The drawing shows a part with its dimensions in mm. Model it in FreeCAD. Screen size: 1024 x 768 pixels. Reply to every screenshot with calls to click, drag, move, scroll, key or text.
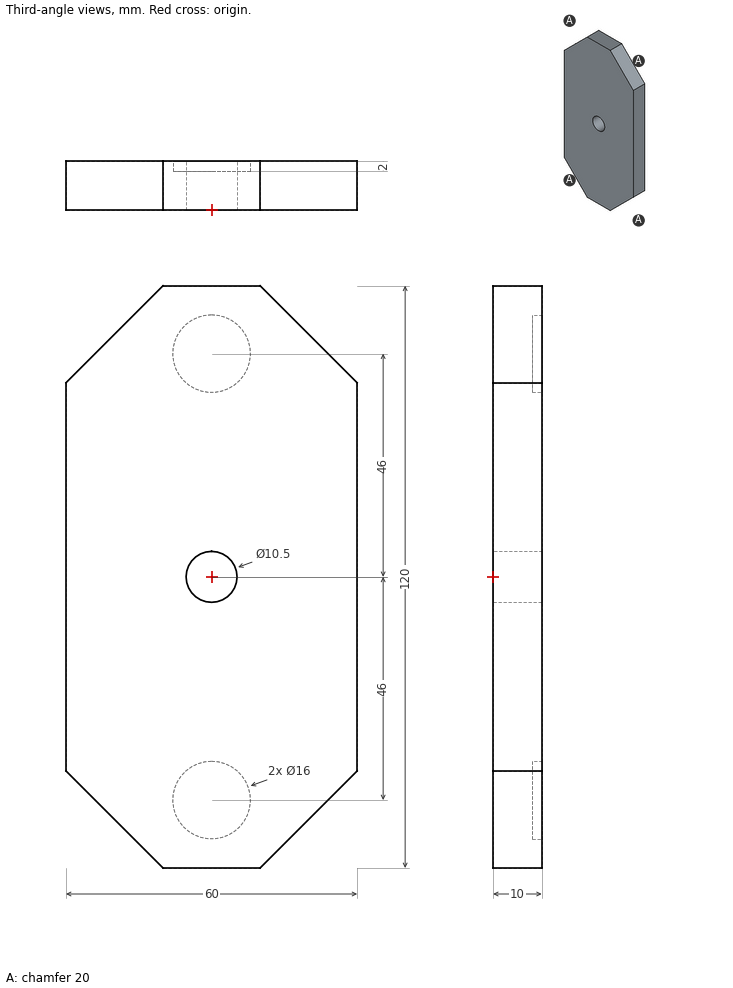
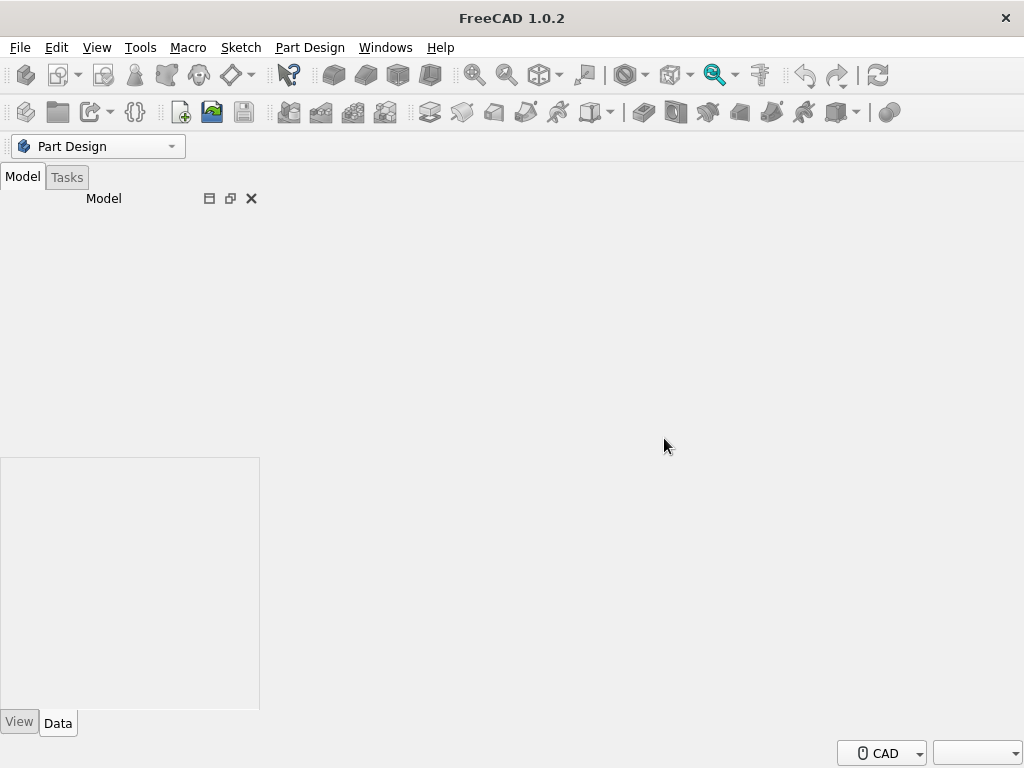
click(180, 112)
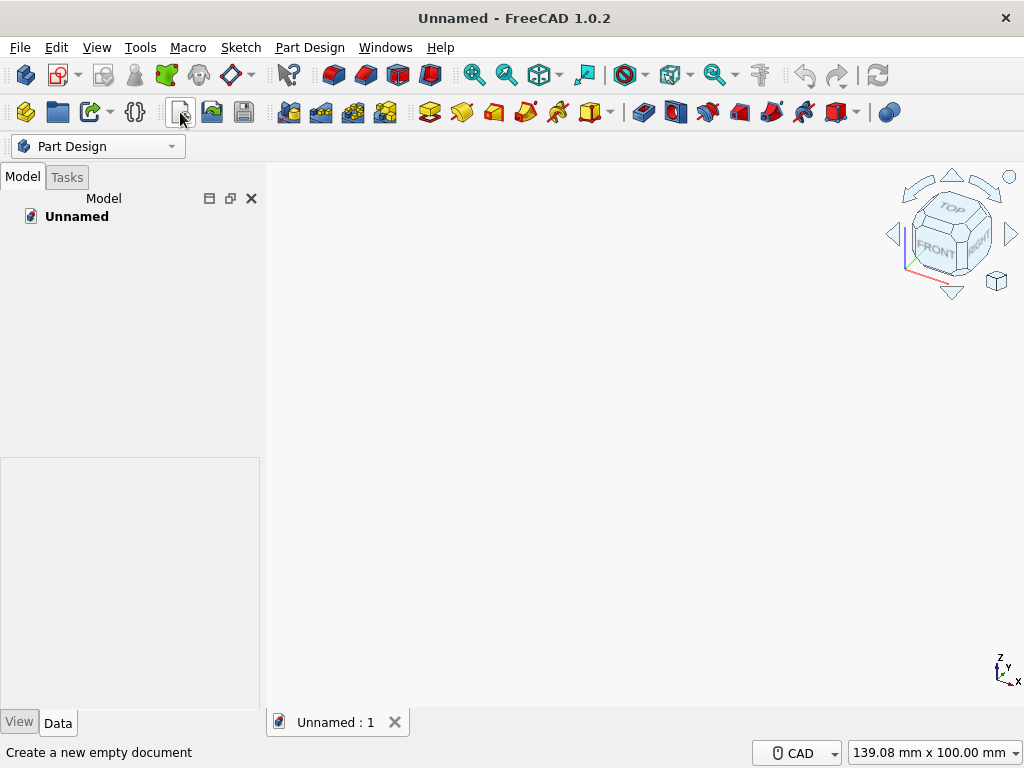
click(58, 76)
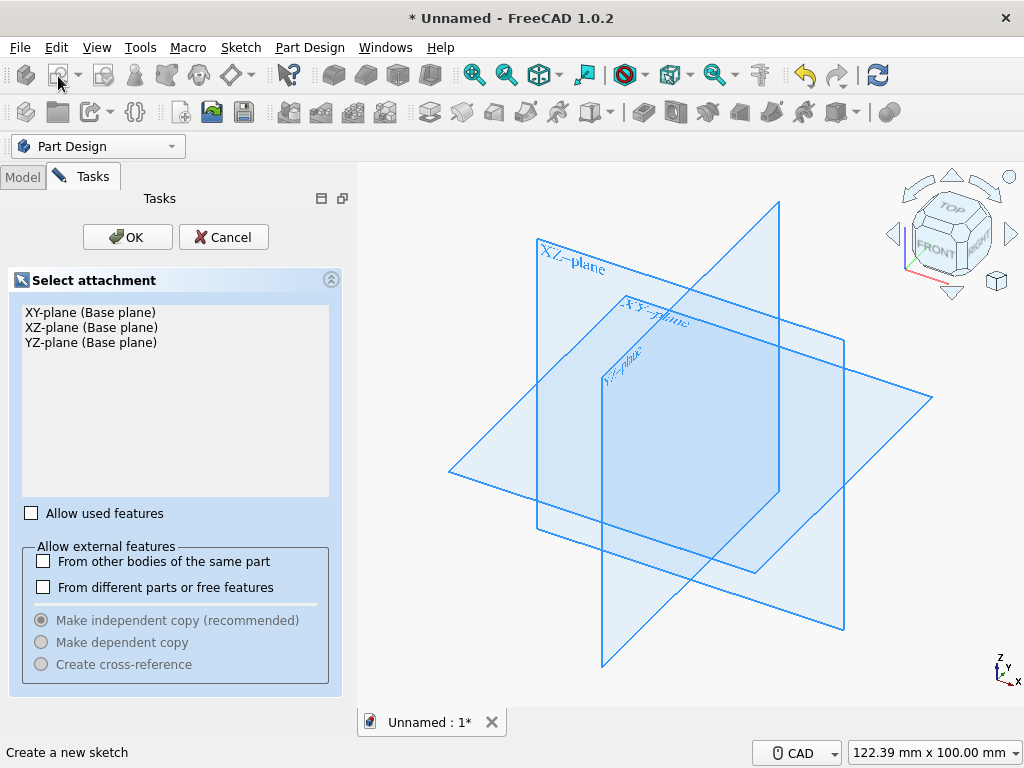
click(82, 328)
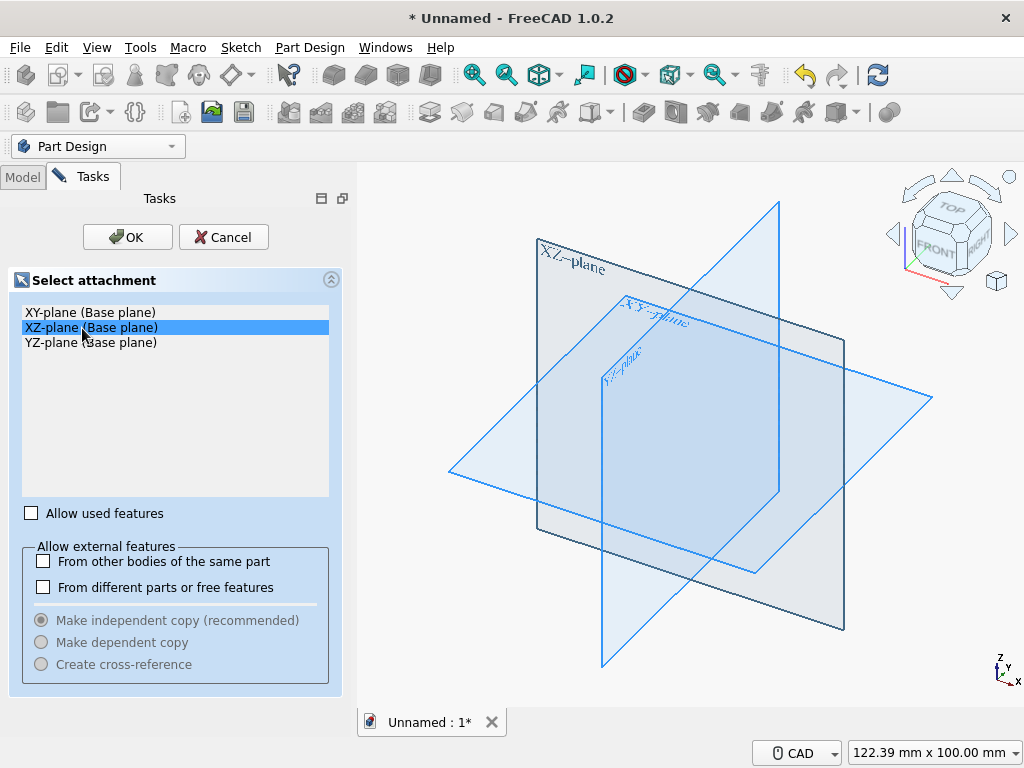
click(128, 237)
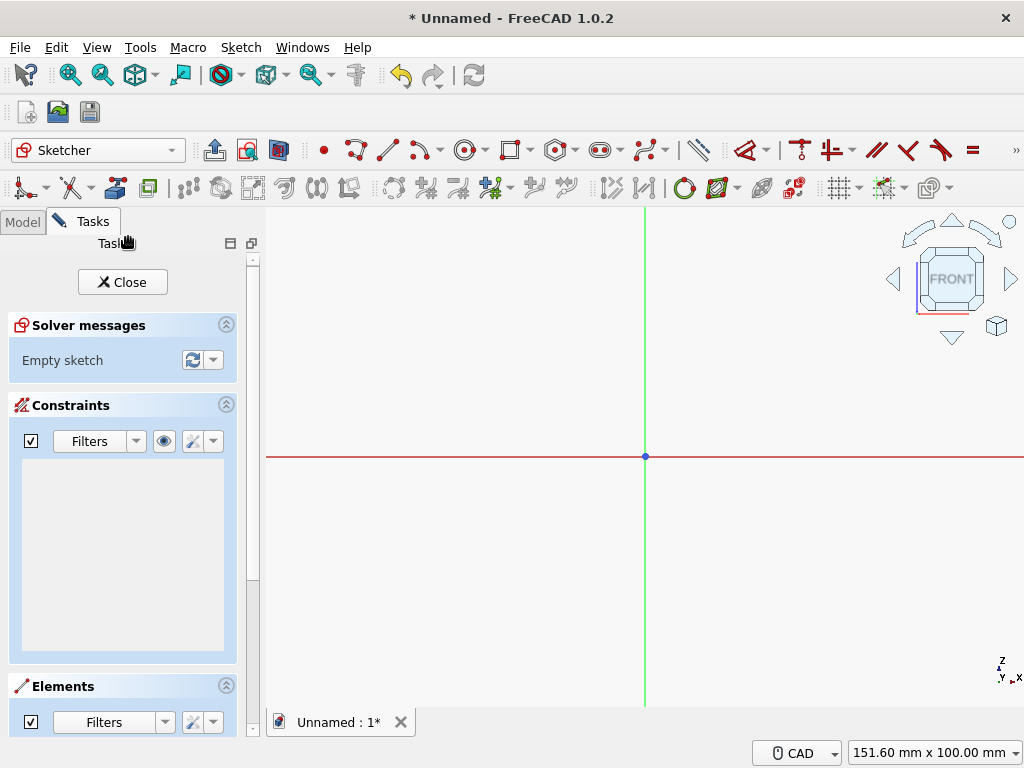
scroll(493, 457, down, 3)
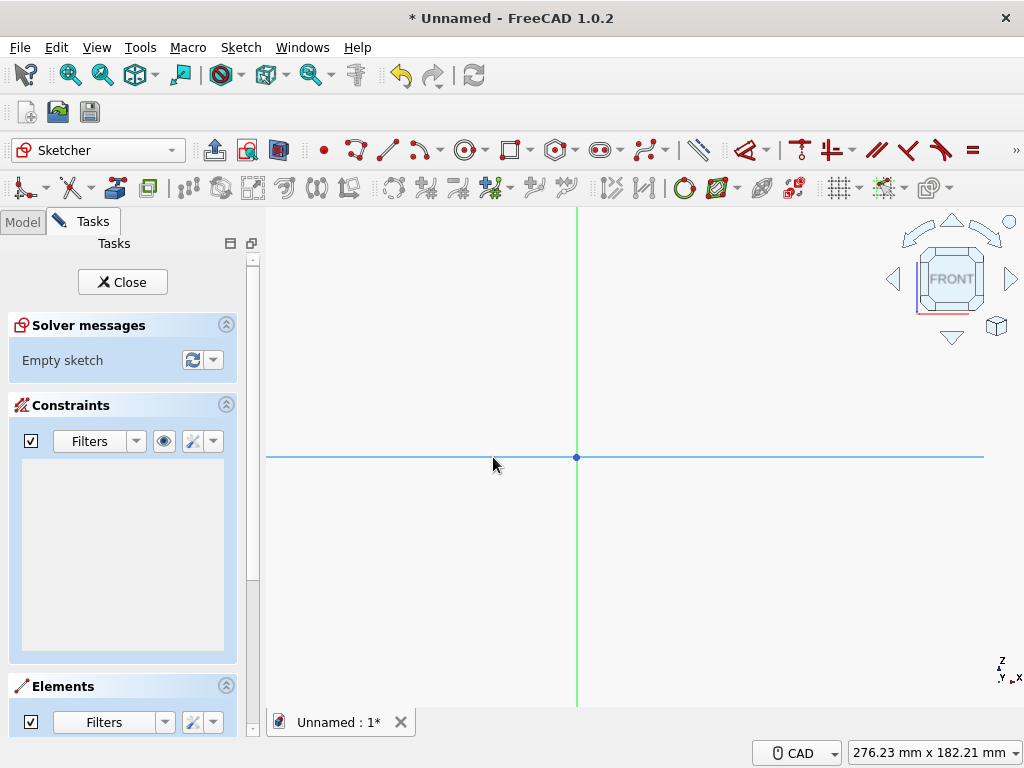
click(532, 150)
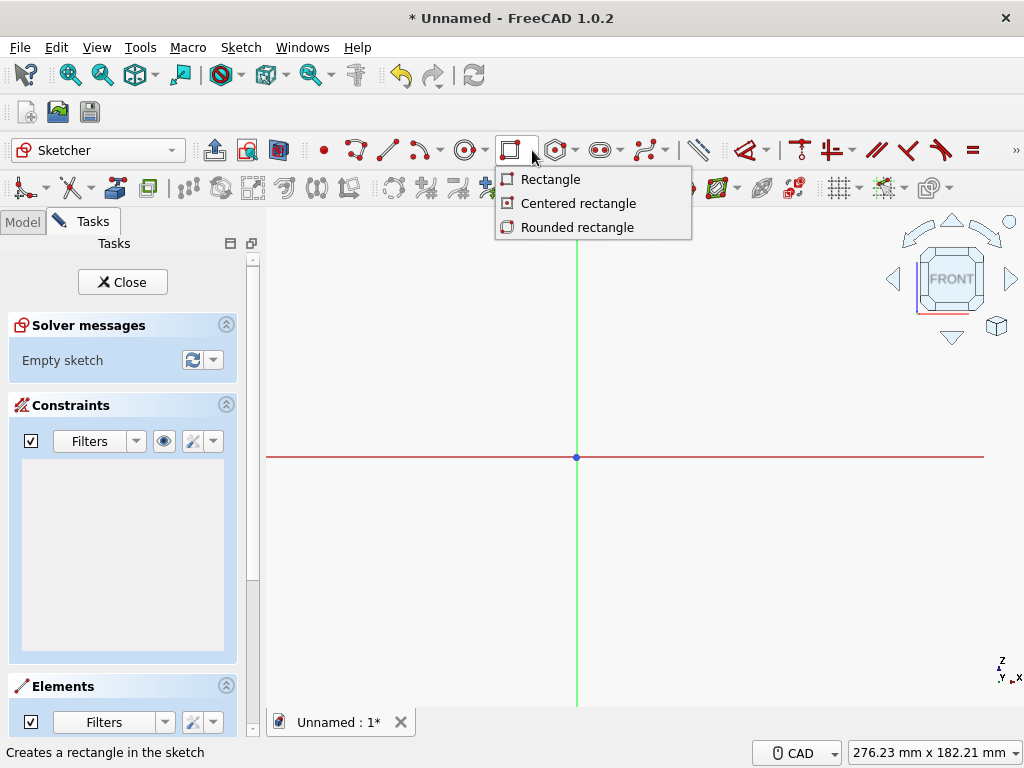
click(594, 203)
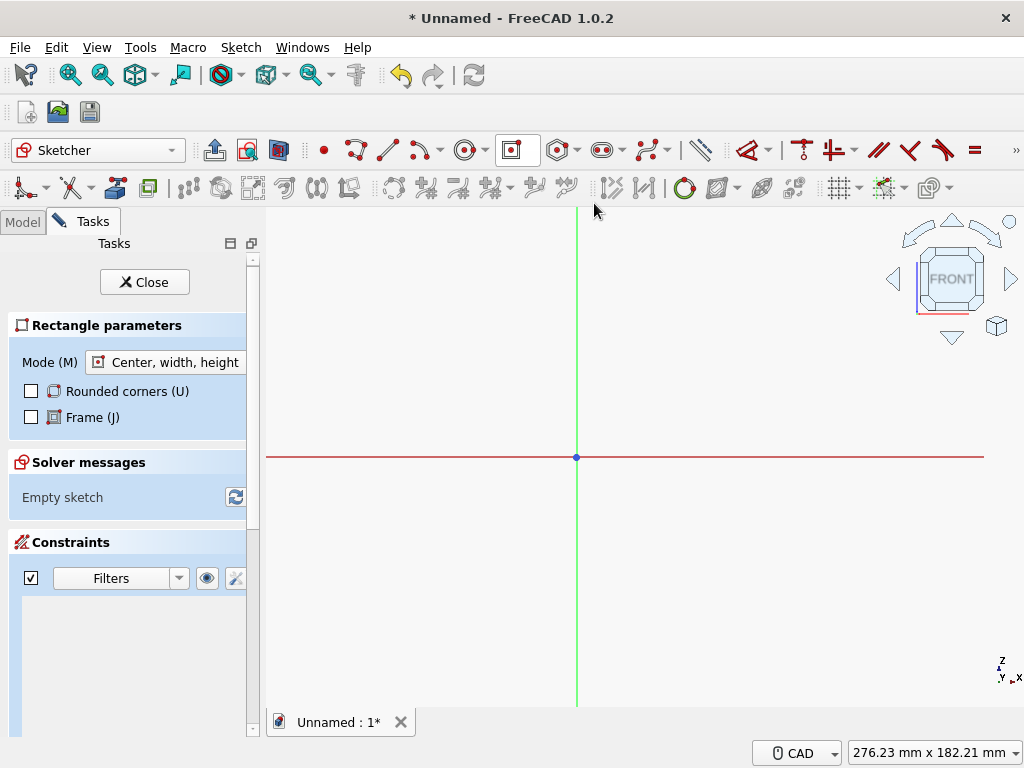
click(577, 457)
click(659, 293)
key(Escape)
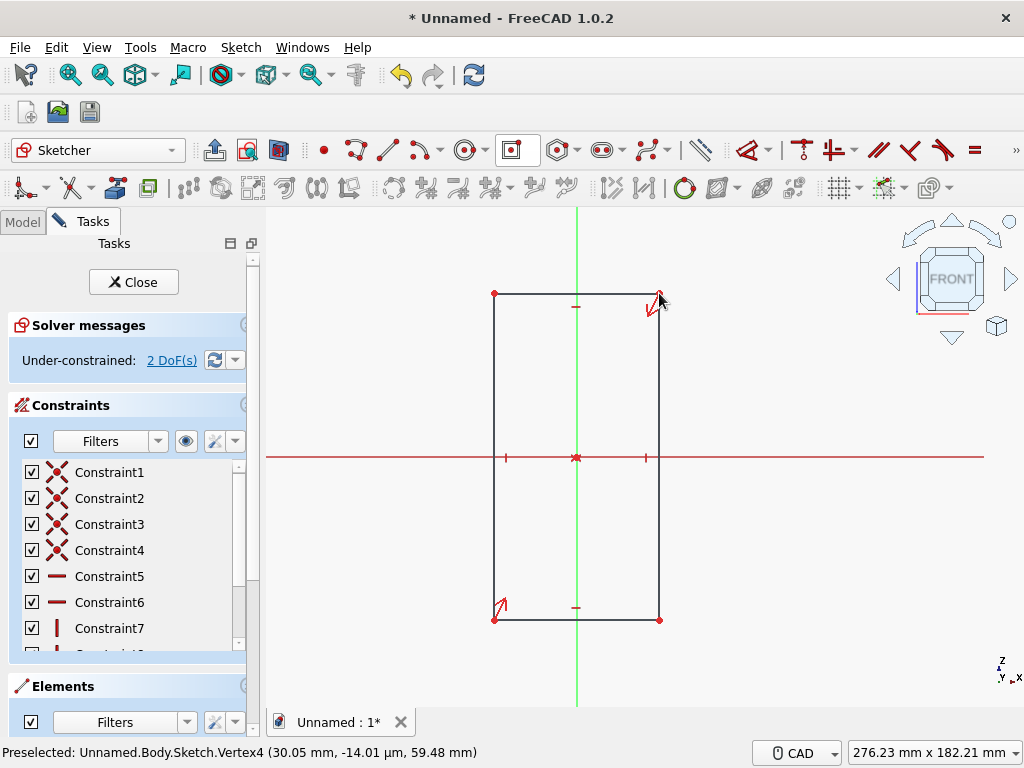
click(748, 150)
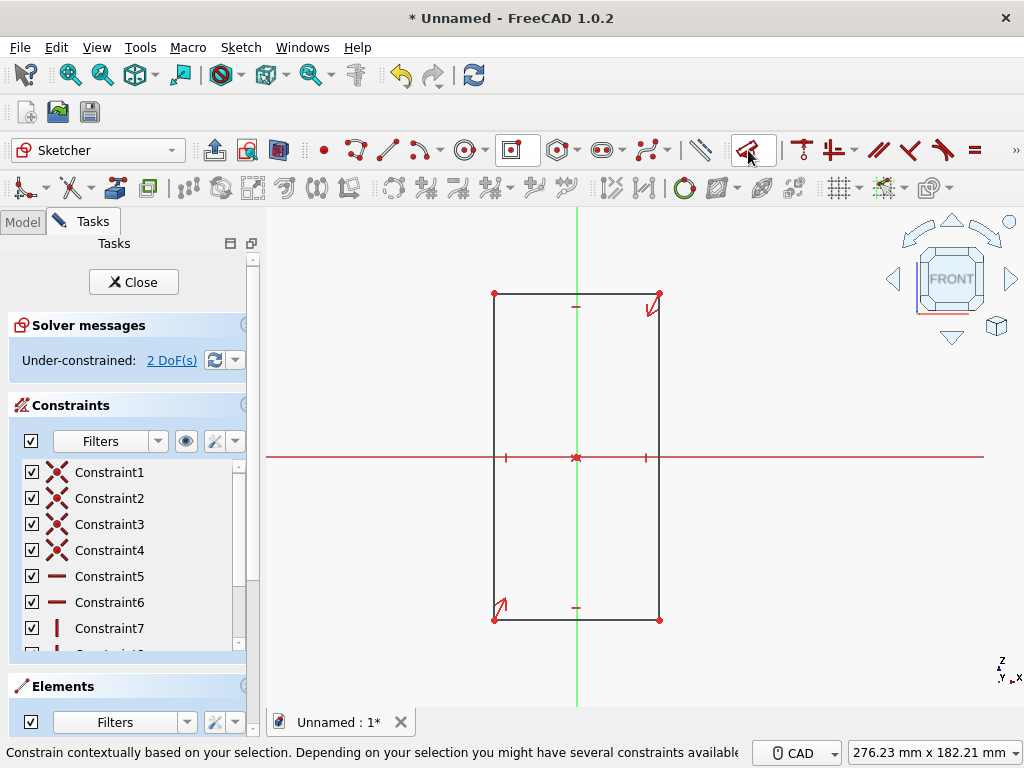
click(544, 620)
click(539, 654)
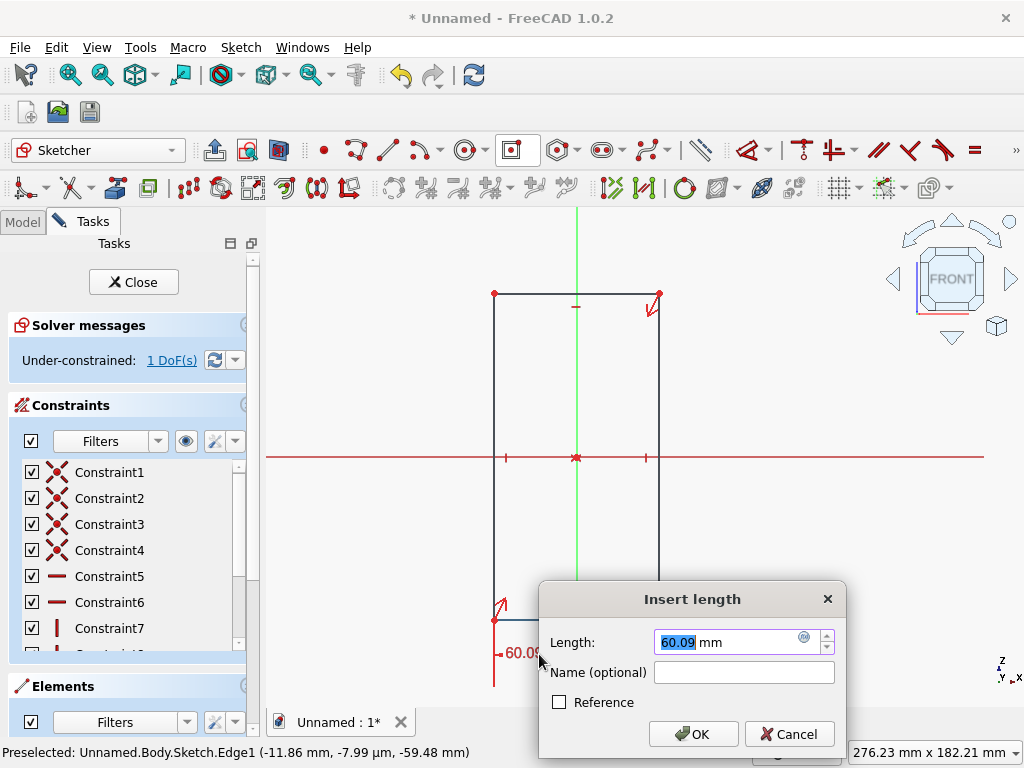
text(60)
key(Return)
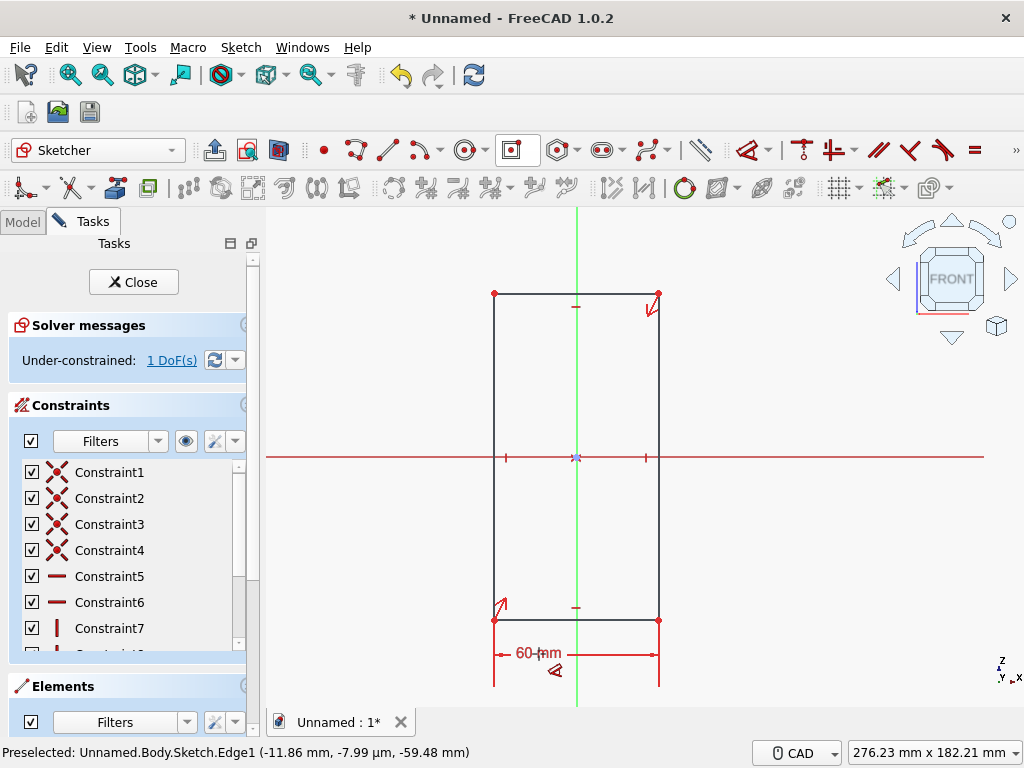
click(659, 523)
click(693, 382)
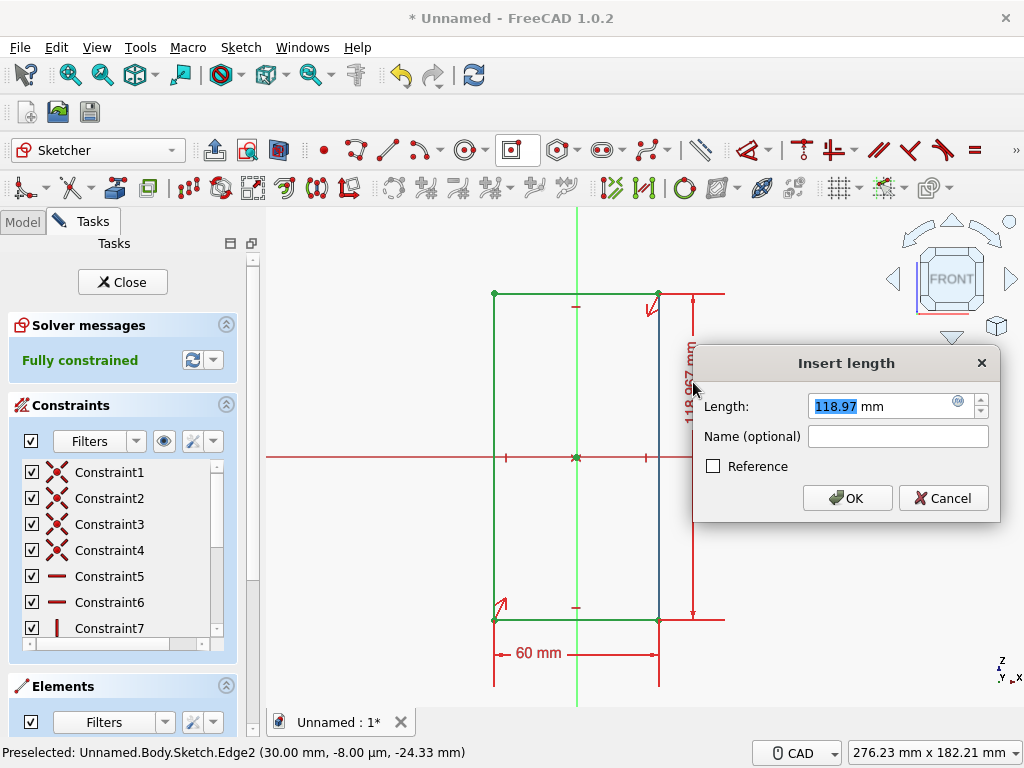
text(120)
key(Return)
key(Escape)